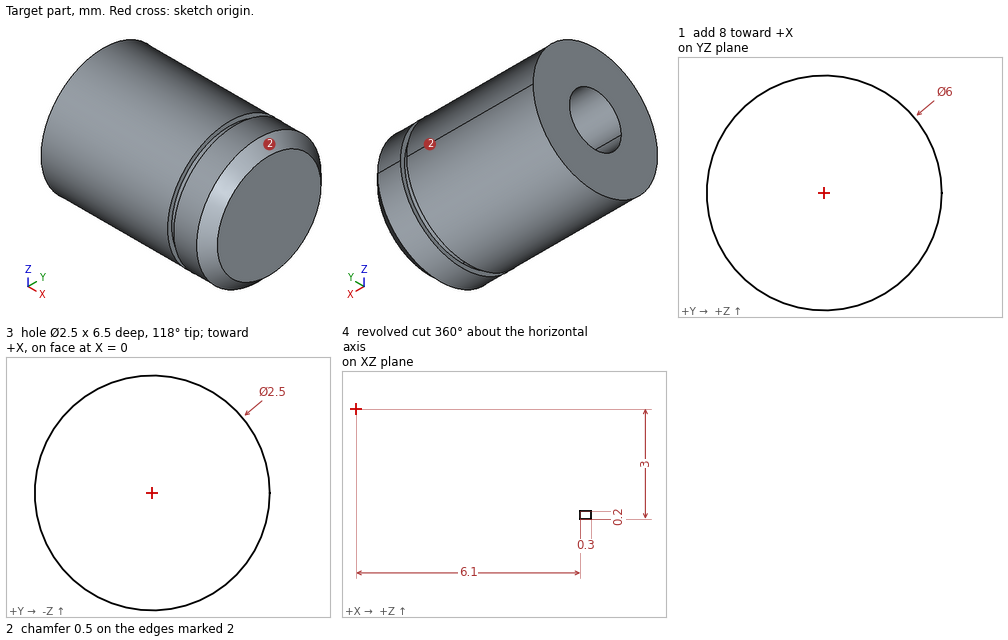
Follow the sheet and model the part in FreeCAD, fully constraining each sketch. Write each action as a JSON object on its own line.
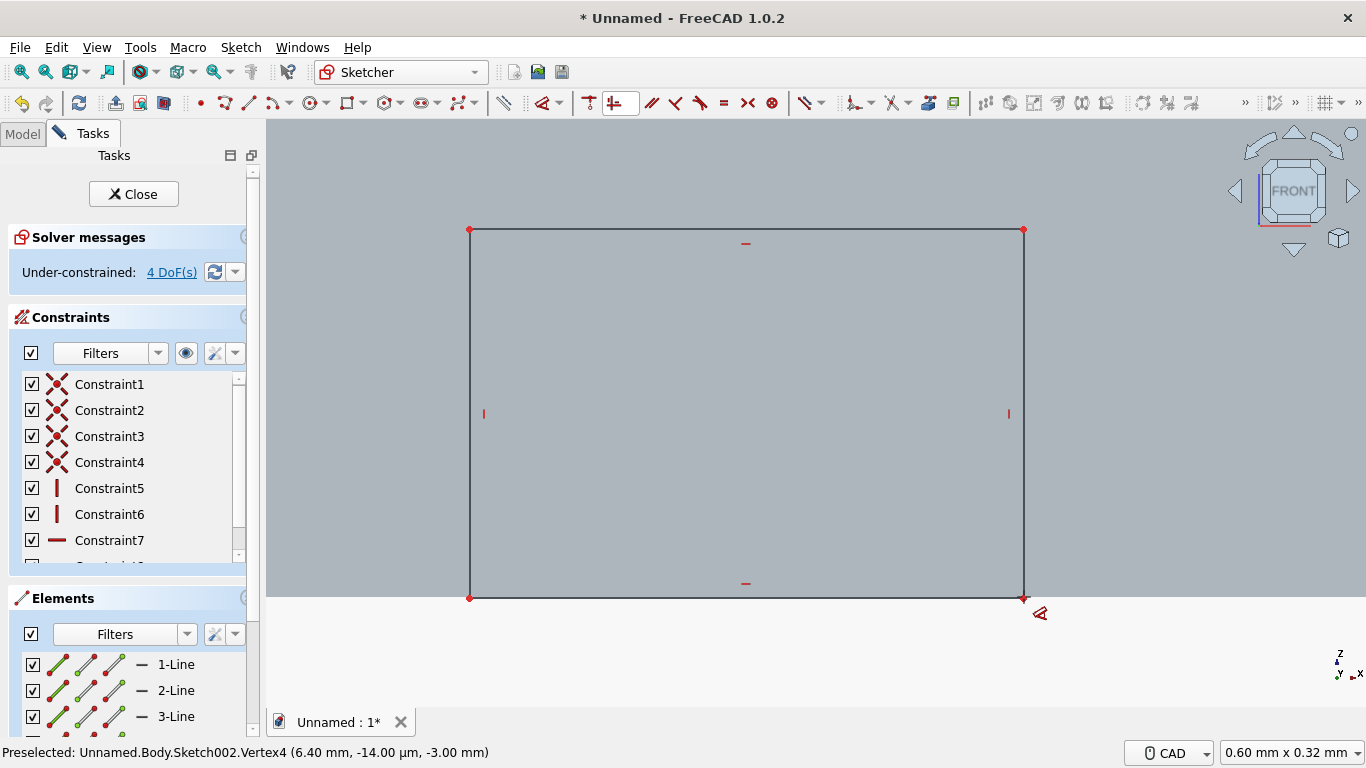
{"action": "left_click", "coordinate": [470, 598]}
{"action": "left_click", "coordinate": [504, 372]}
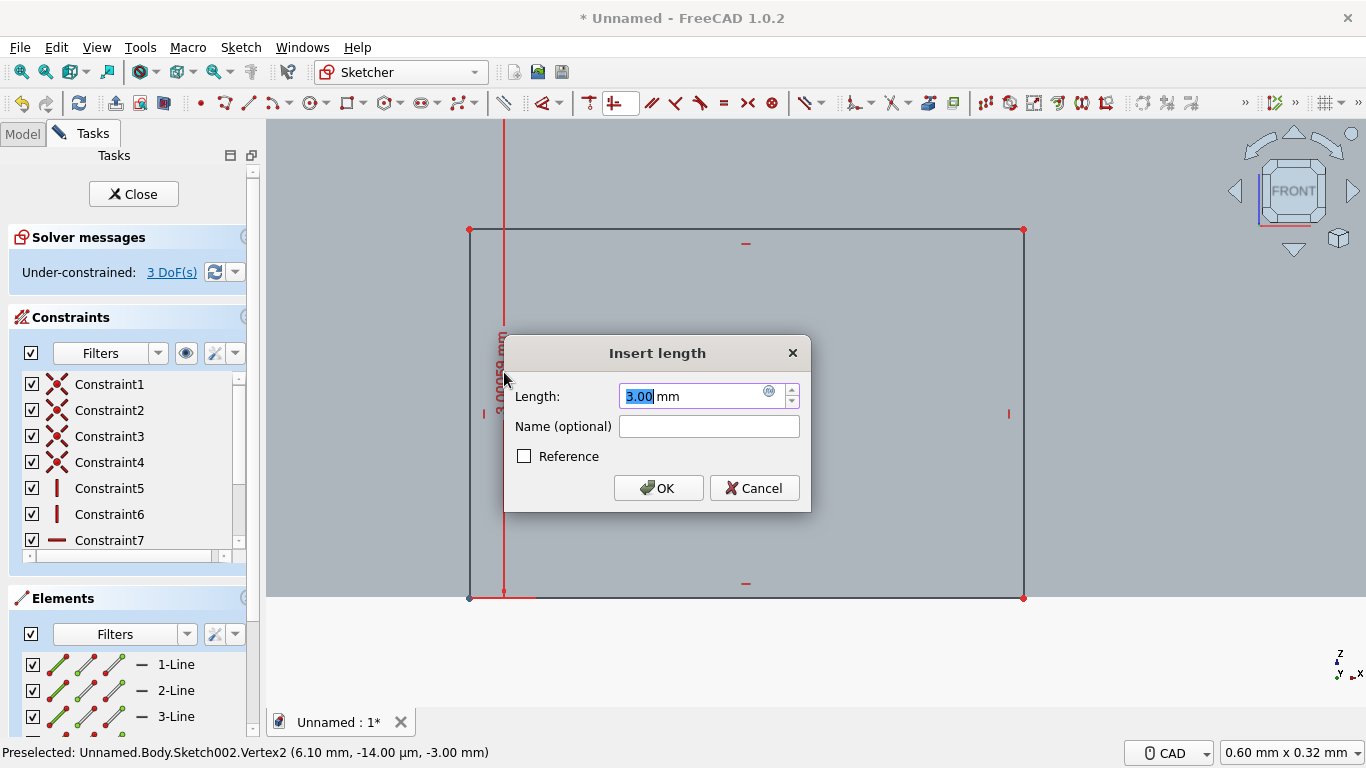
{"action": "type", "text": "3"}
{"action": "key", "text": "Return"}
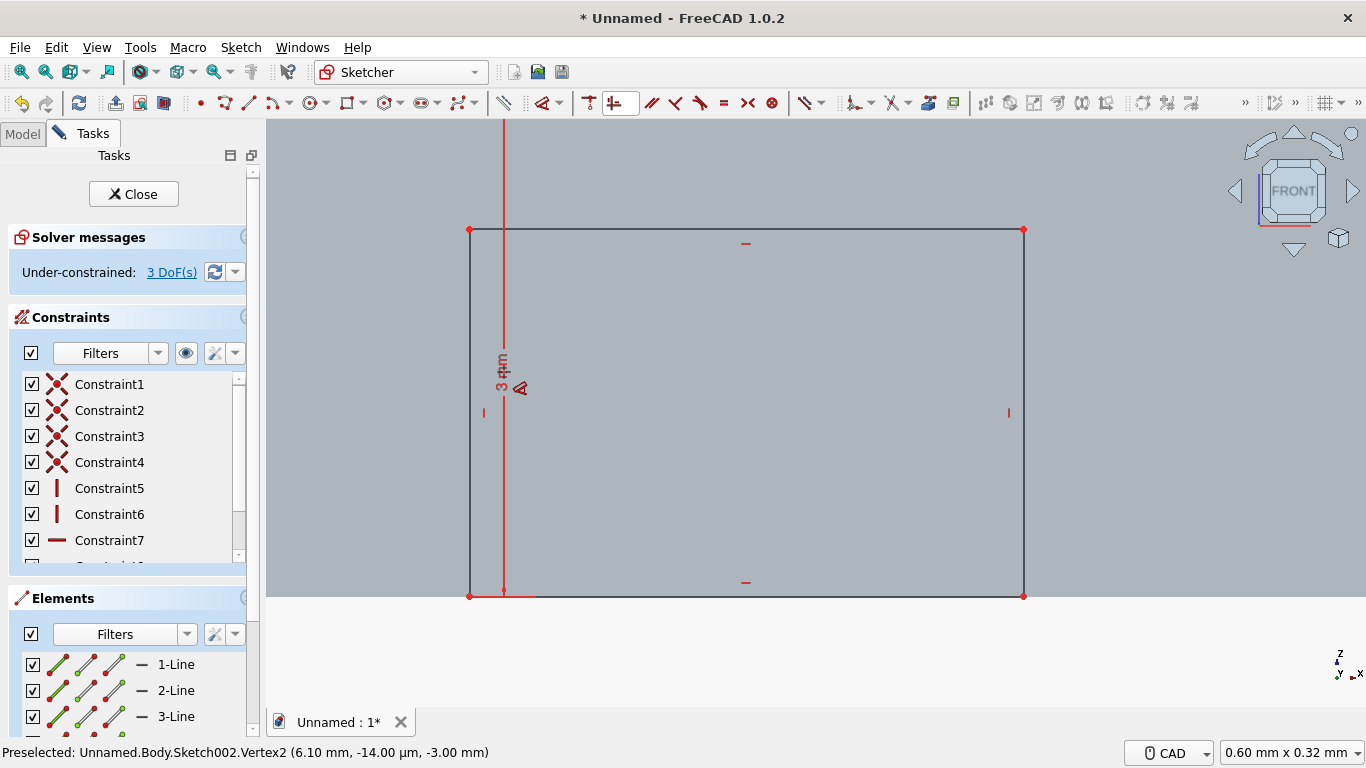
{"action": "left_click", "coordinate": [470, 339]}
{"action": "left_click", "coordinate": [436, 413]}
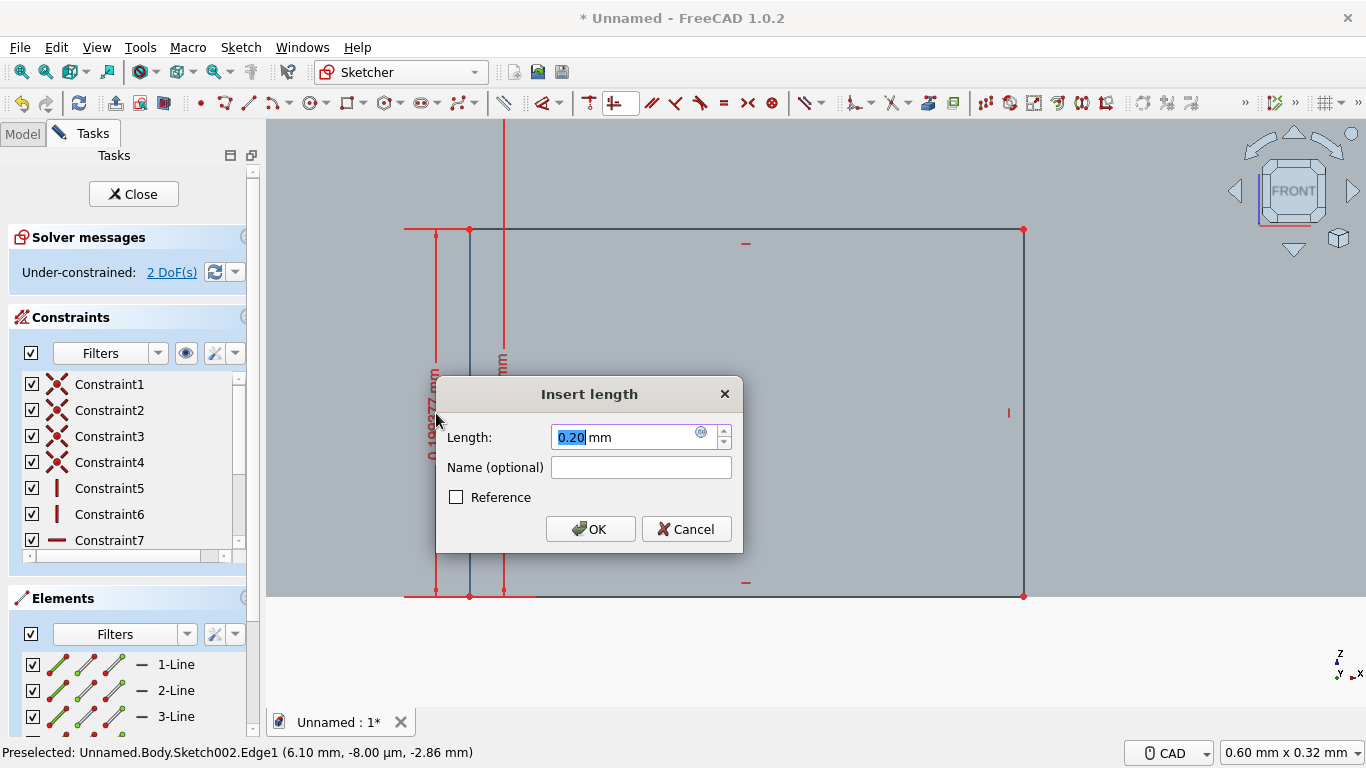
{"action": "type", "text": "0.2"}
{"action": "key", "text": "Return"}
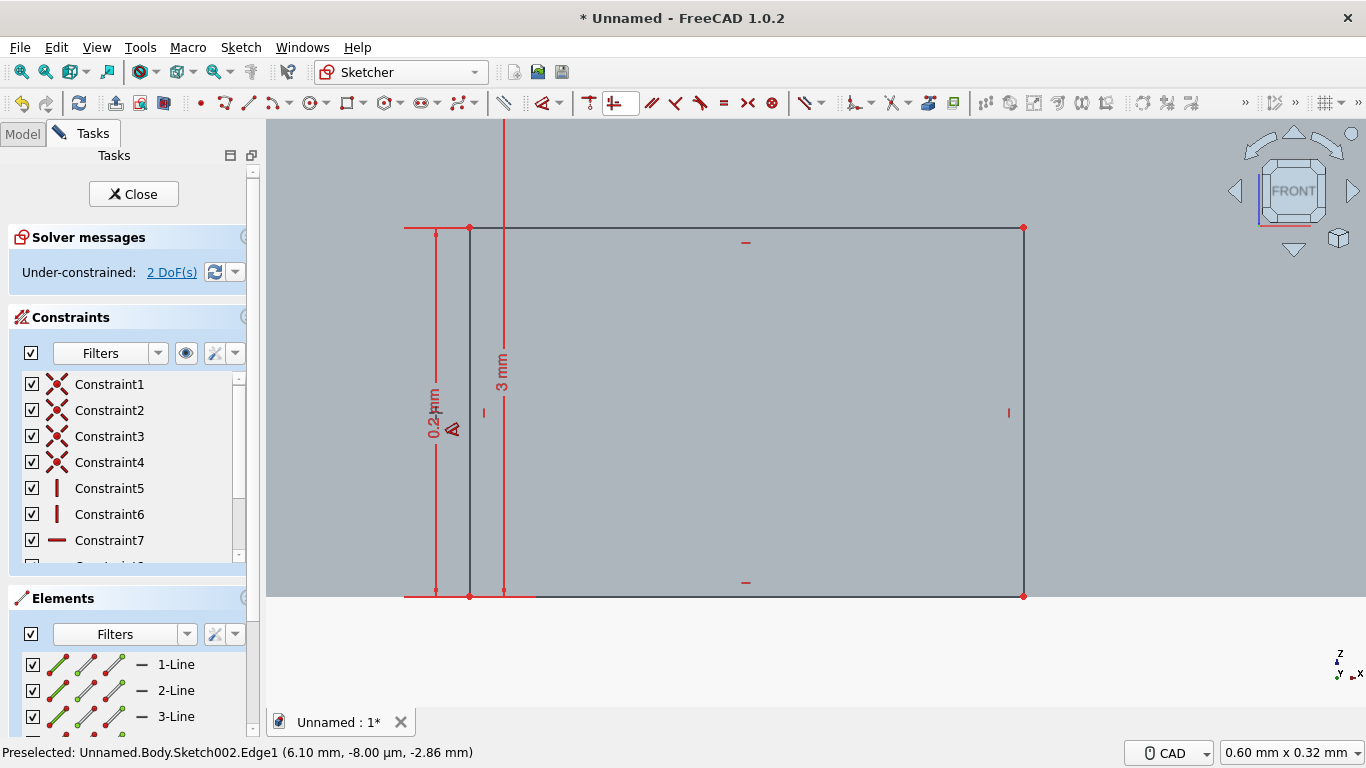
{"action": "left_click", "coordinate": [636, 597]}
{"action": "left_click", "coordinate": [747, 631]}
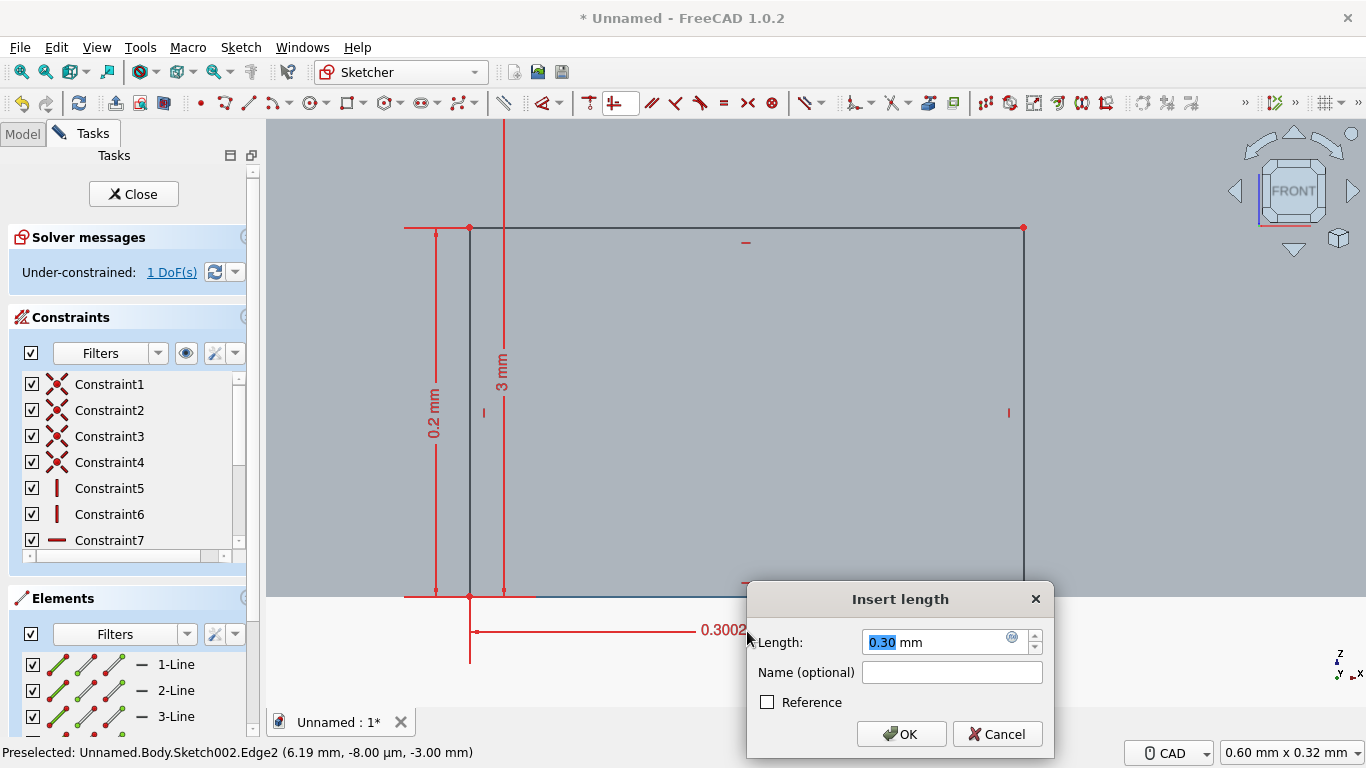
{"action": "type", "text": "0.3"}
{"action": "key", "text": "Return"}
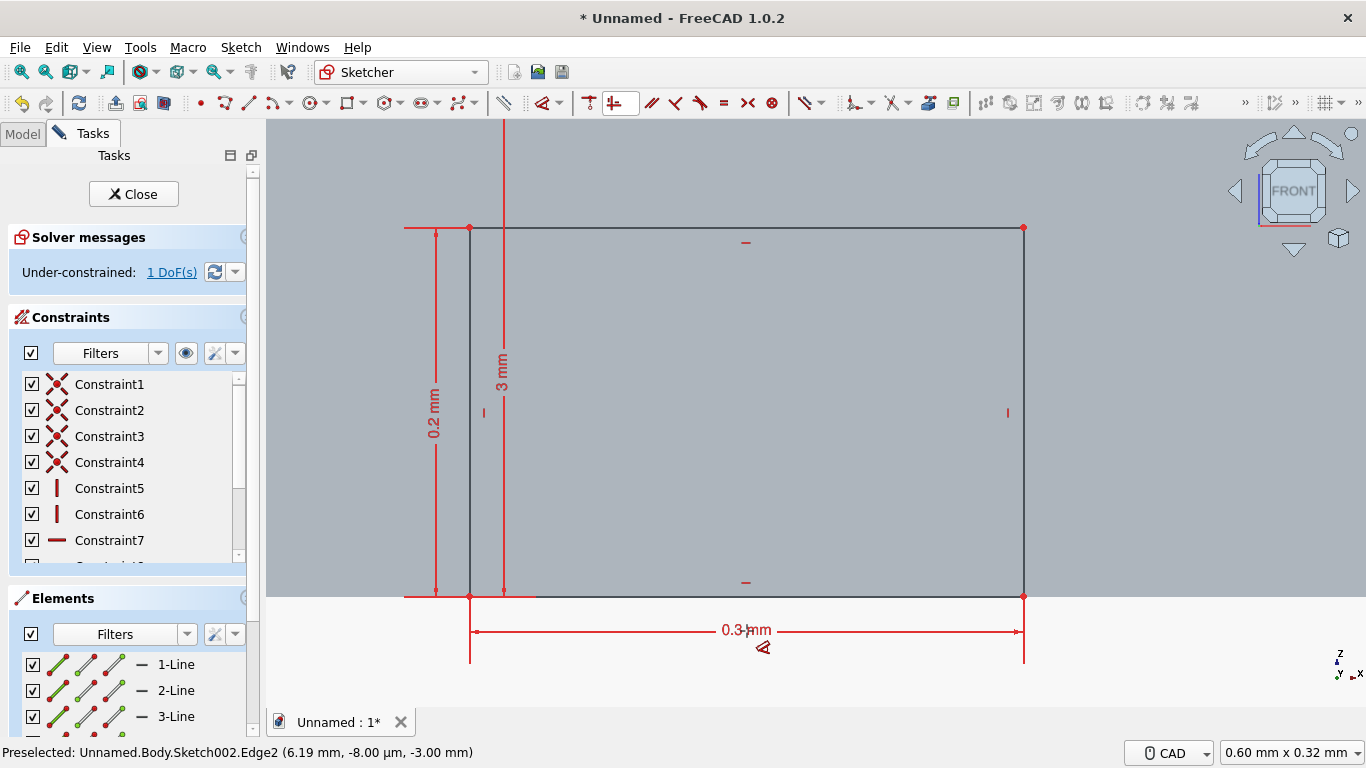
{"action": "left_click", "coordinate": [470, 228]}
{"action": "left_click", "coordinate": [382, 262]}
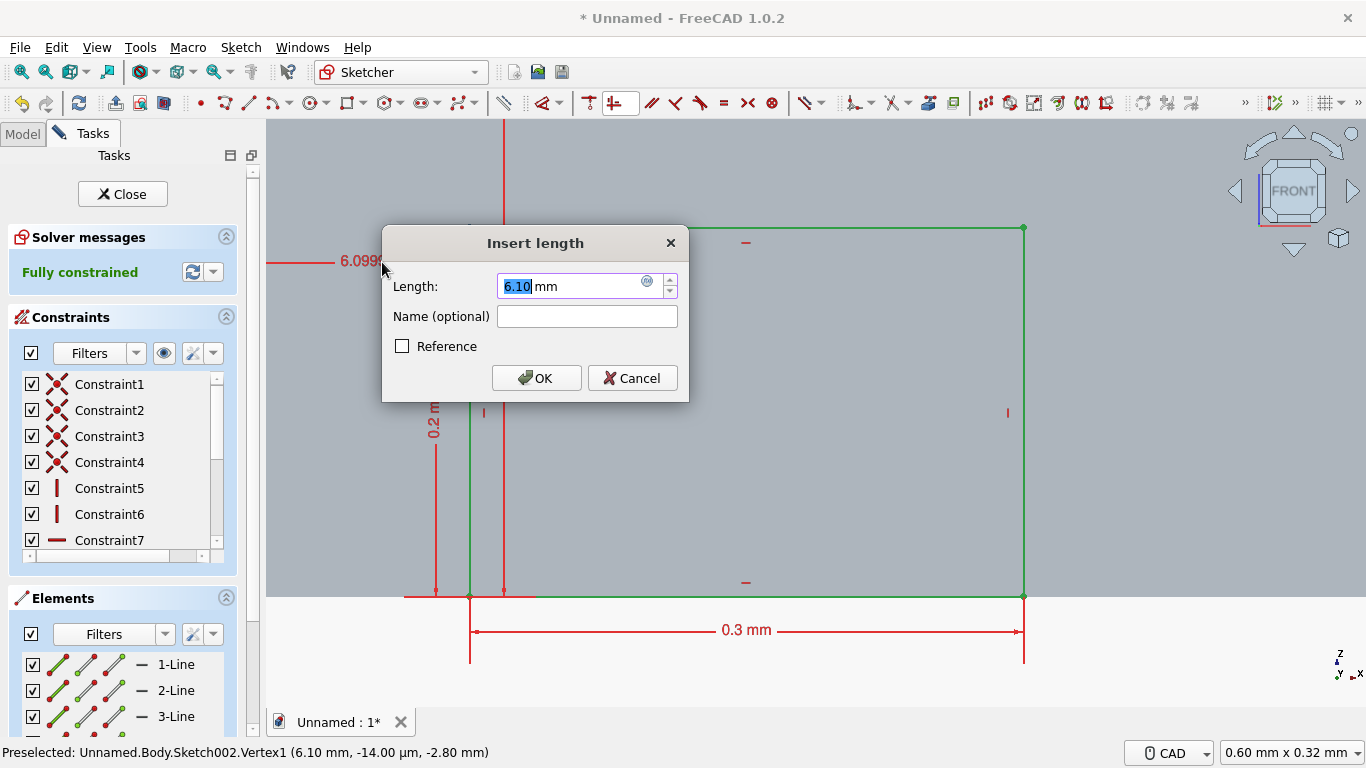
{"action": "type", "text": "6.1"}
{"action": "key", "text": "Return"}
{"action": "key", "text": "Escape"}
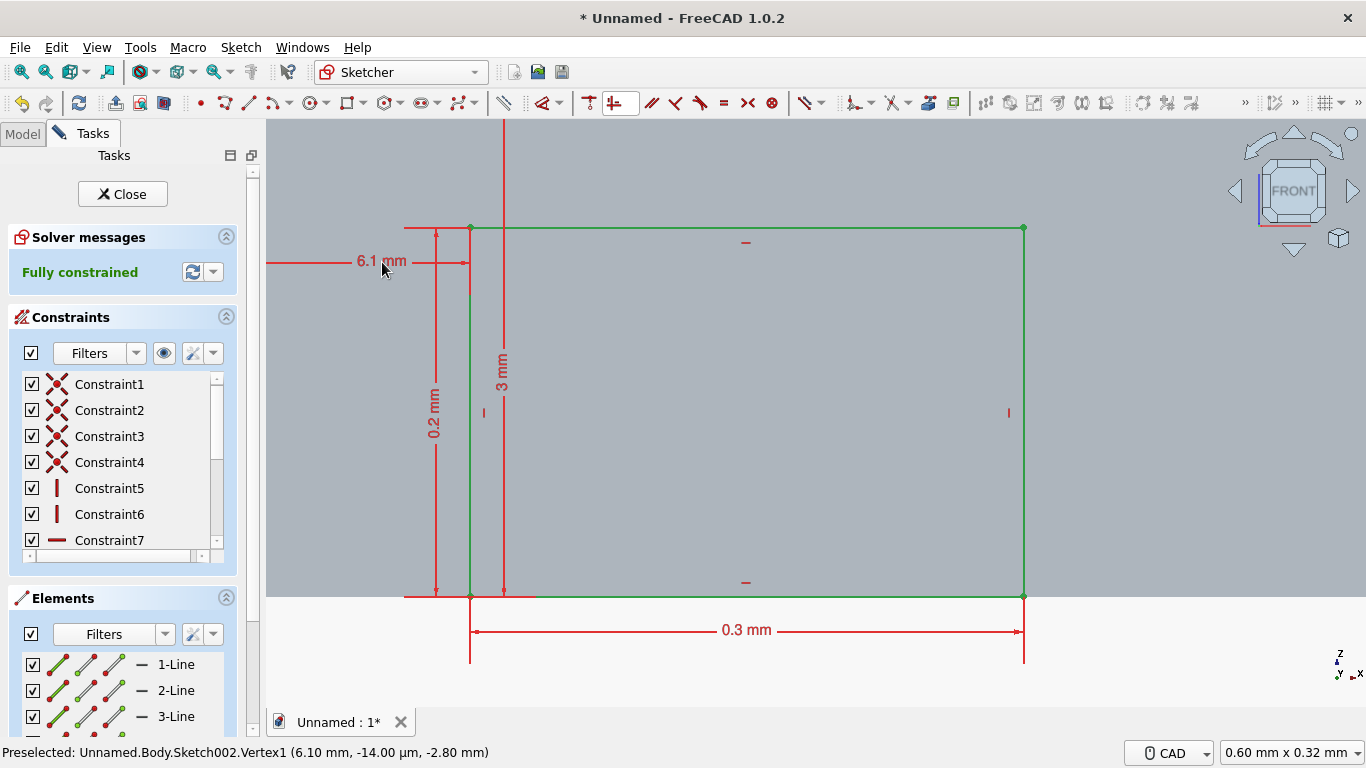
{"action": "left_click", "coordinate": [123, 194]}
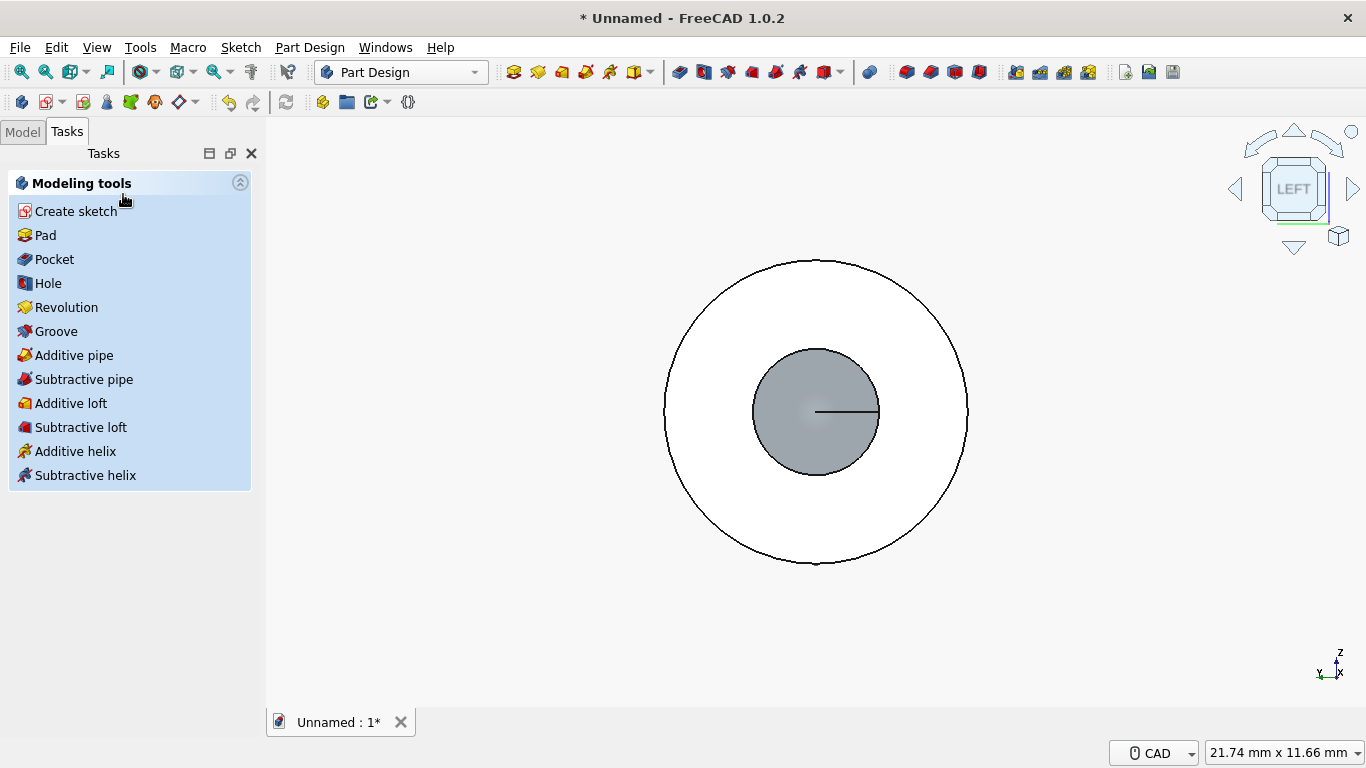
{"action": "left_click", "coordinate": [728, 72]}